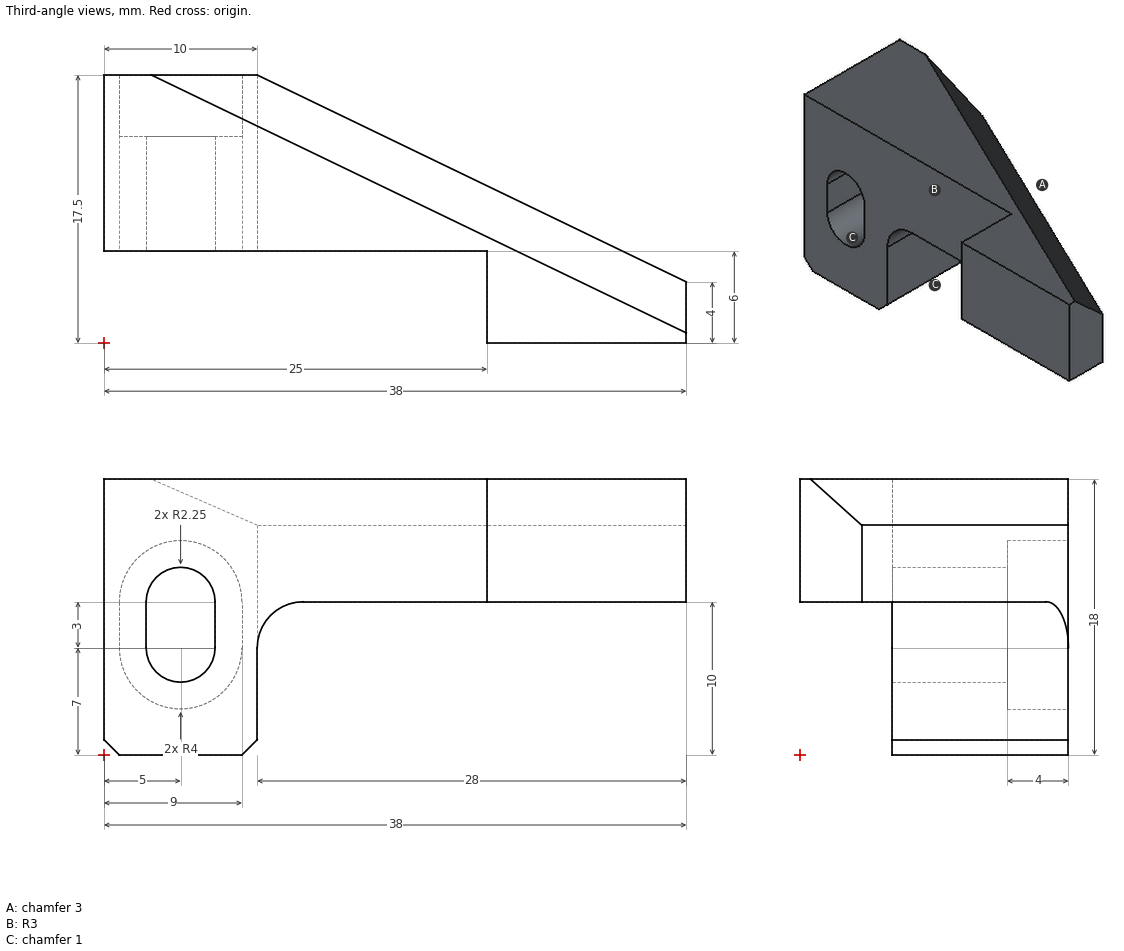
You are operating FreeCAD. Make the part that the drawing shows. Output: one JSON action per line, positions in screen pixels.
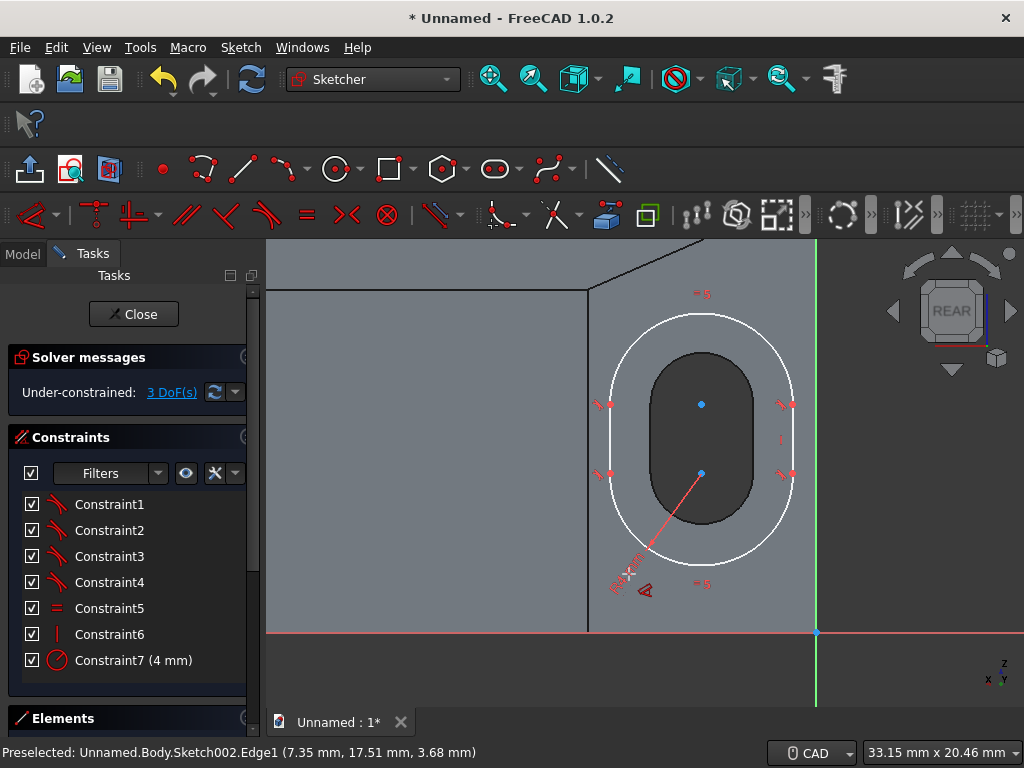
{"action": "left_click", "coordinate": [610, 453]}
{"action": "left_click", "coordinate": [576, 440]}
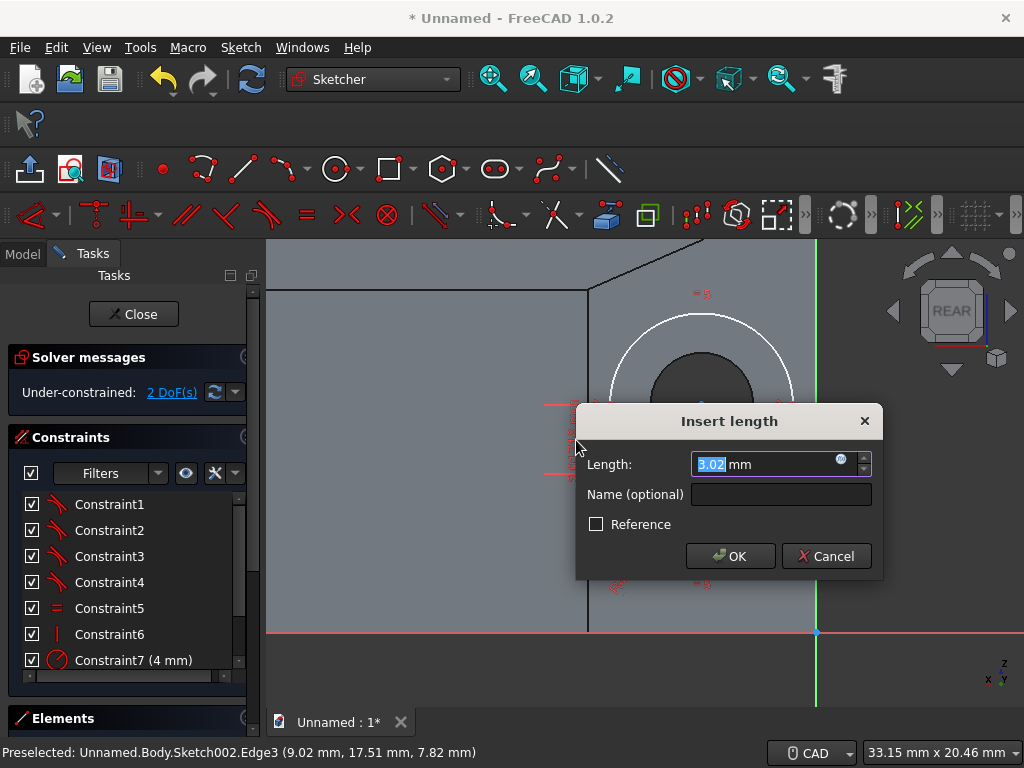
{"action": "type", "text": "3"}
{"action": "key", "text": "Return"}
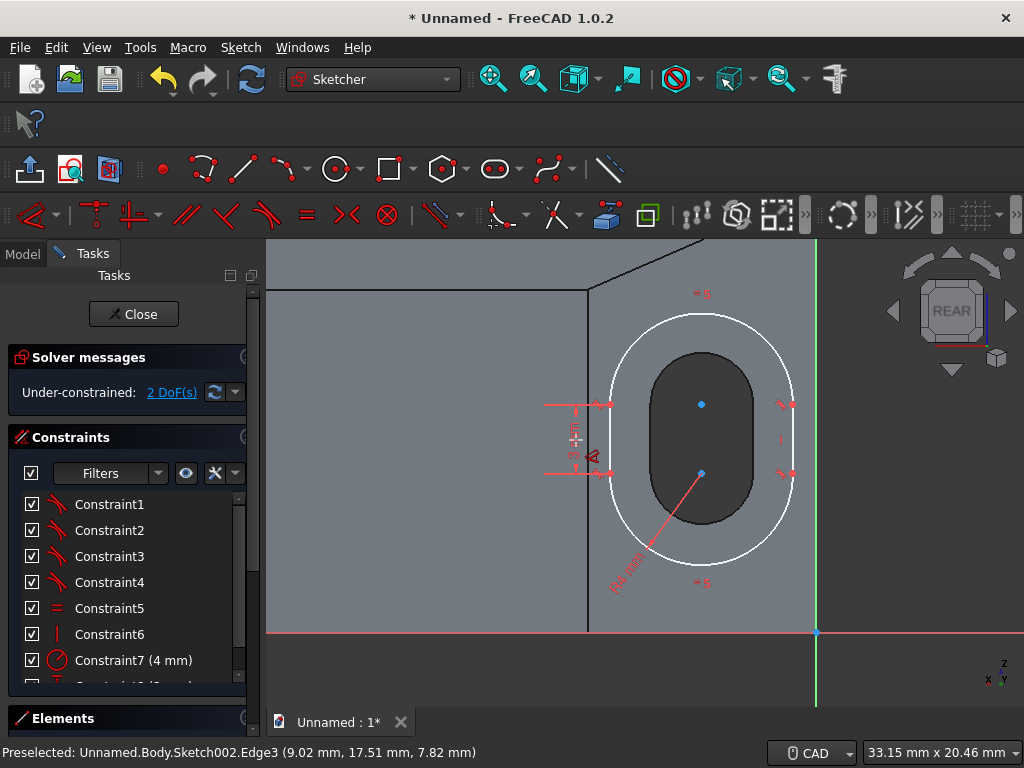
{"action": "left_click", "coordinate": [610, 474]}
{"action": "left_click", "coordinate": [713, 667]}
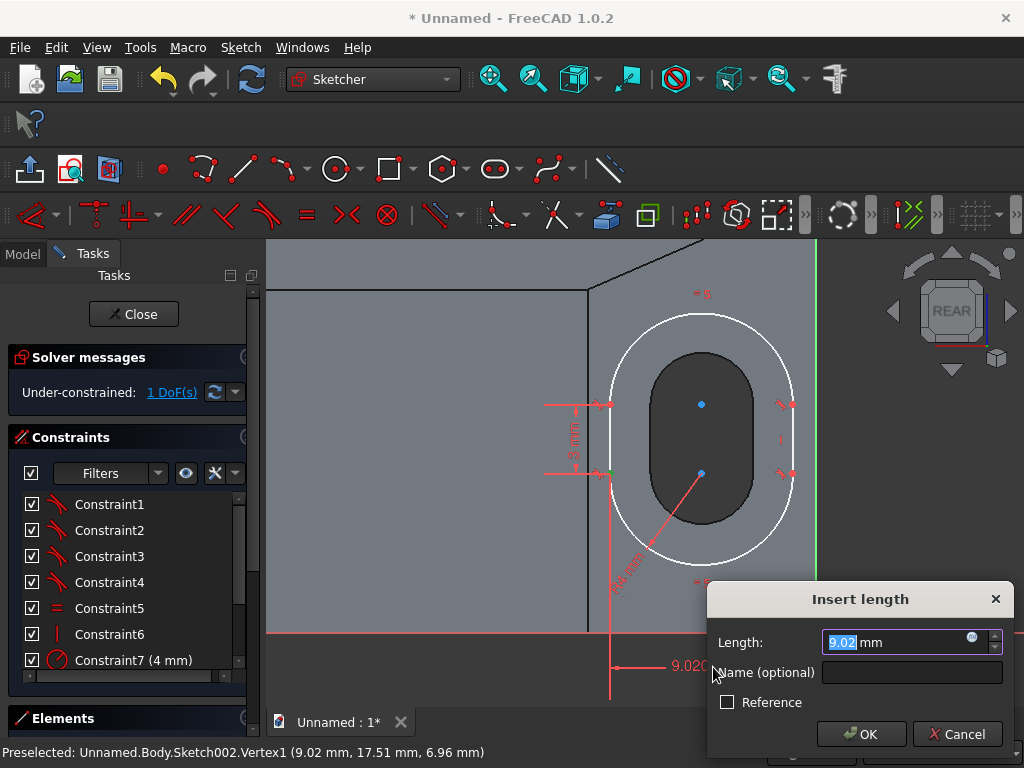
{"action": "type", "text": "9"}
{"action": "key", "text": "Return"}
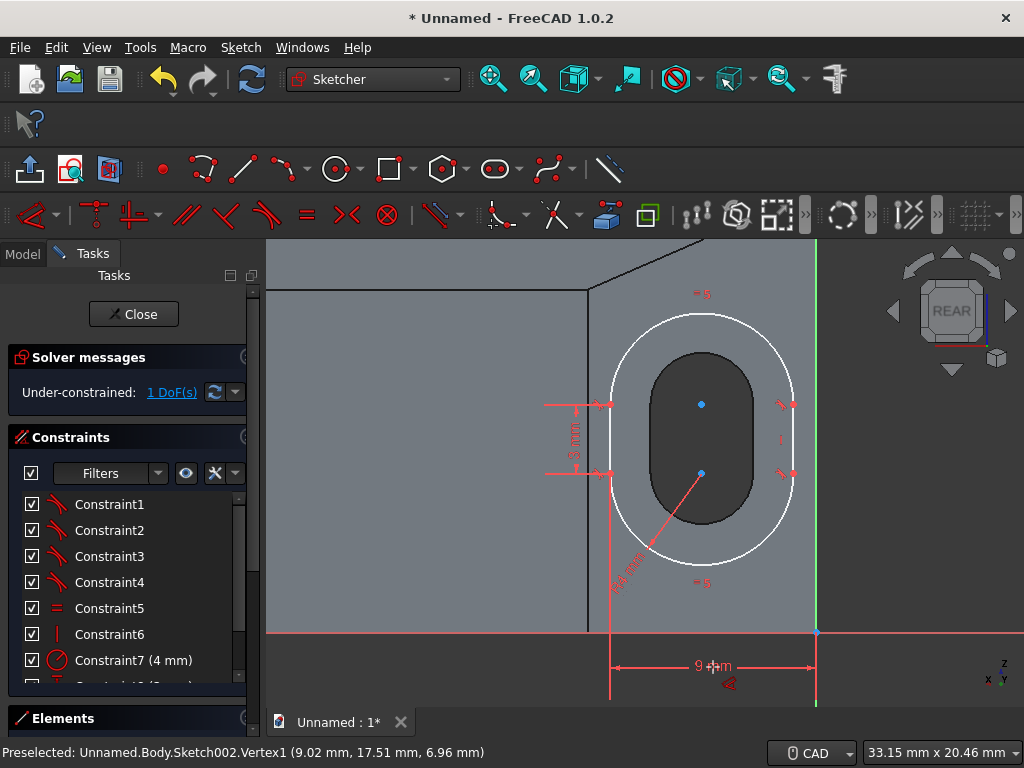
{"action": "left_click", "coordinate": [610, 474]}
{"action": "left_click", "coordinate": [850, 553]}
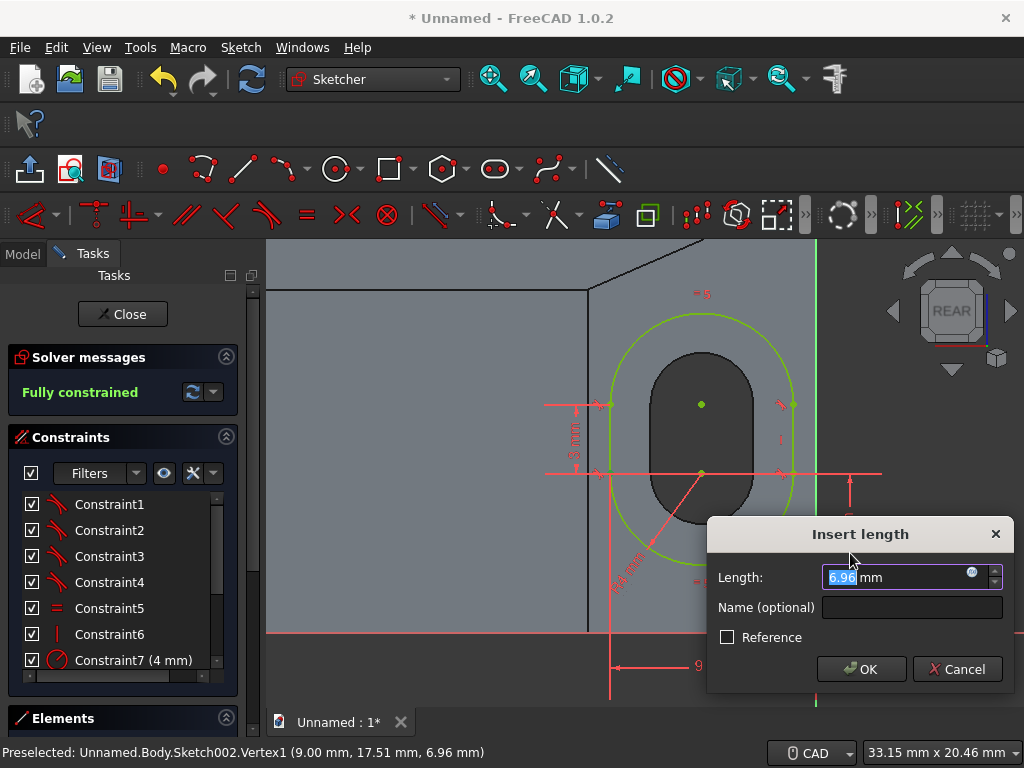
{"action": "type", "text": "7"}
{"action": "key", "text": "Return"}
{"action": "key", "text": "Escape"}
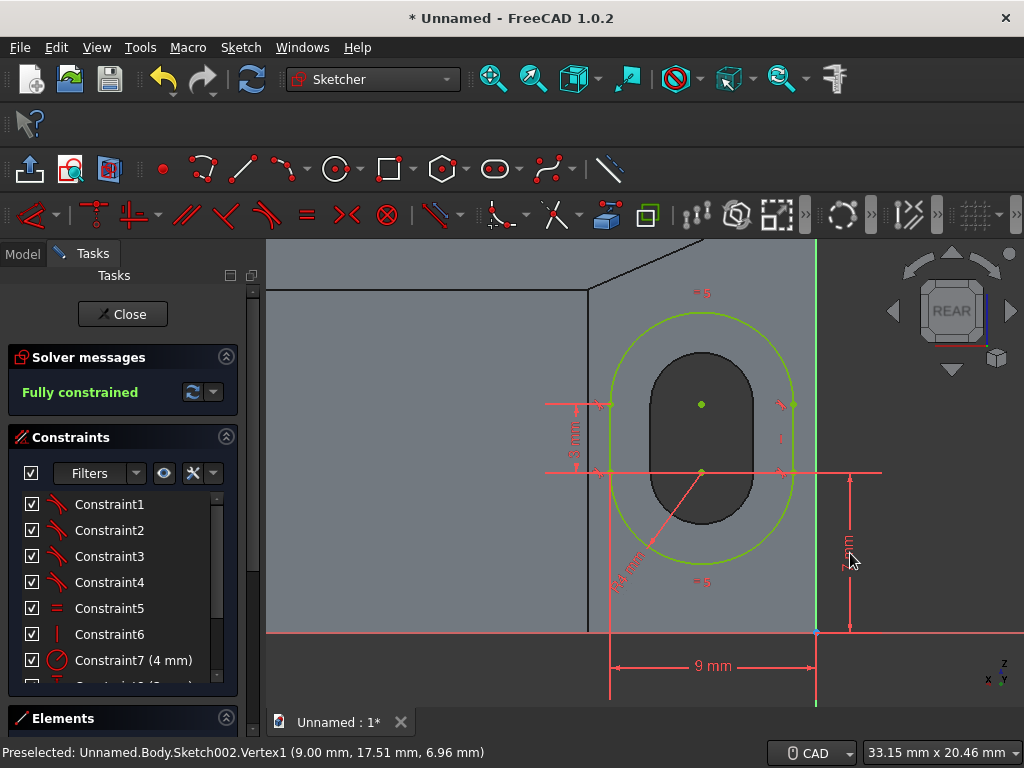
{"action": "left_click", "coordinate": [123, 314]}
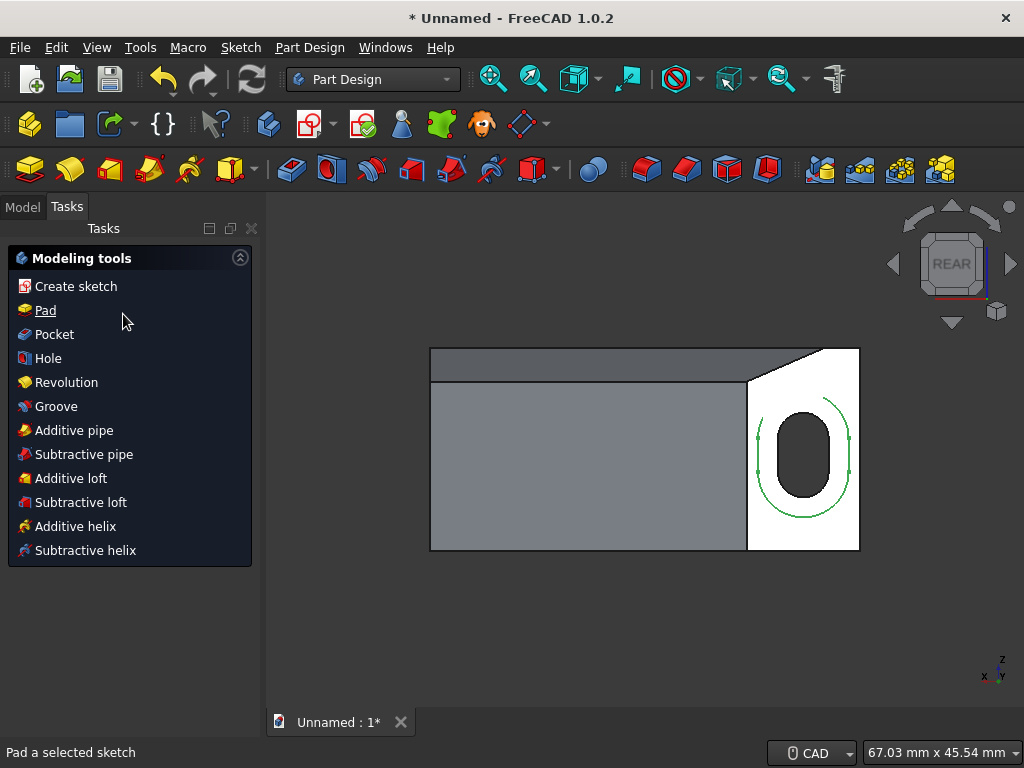
{"action": "left_click", "coordinate": [292, 170]}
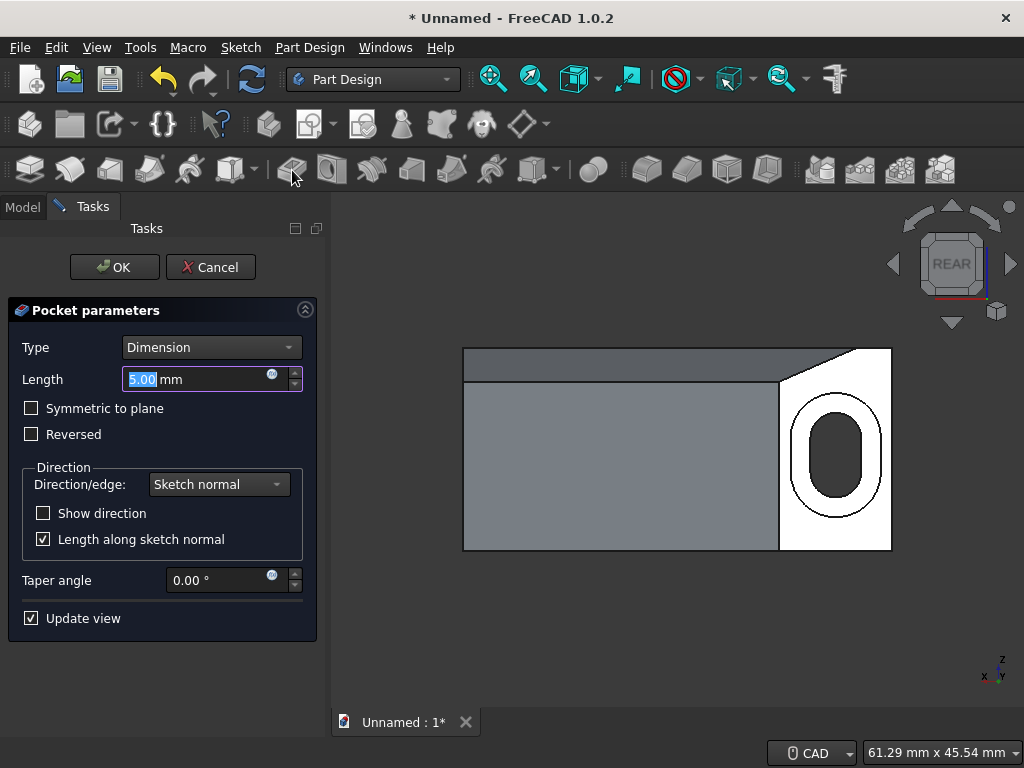
{"action": "type", "text": "4"}
{"action": "key", "text": "Tab"}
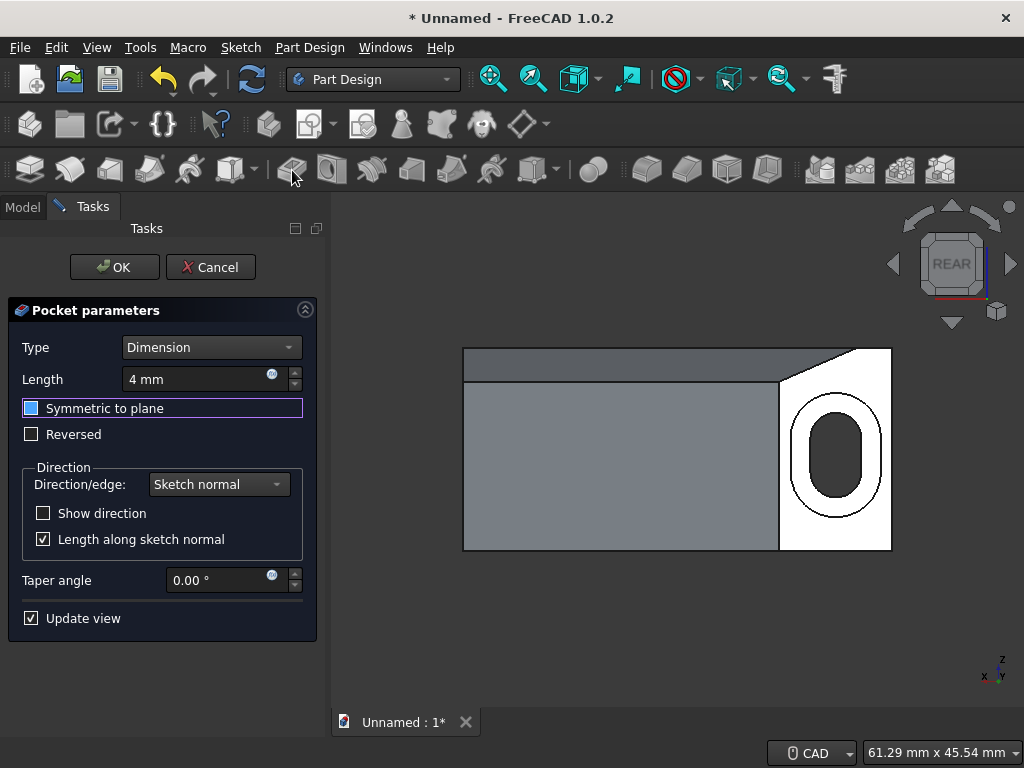
{"action": "left_click", "coordinate": [115, 267]}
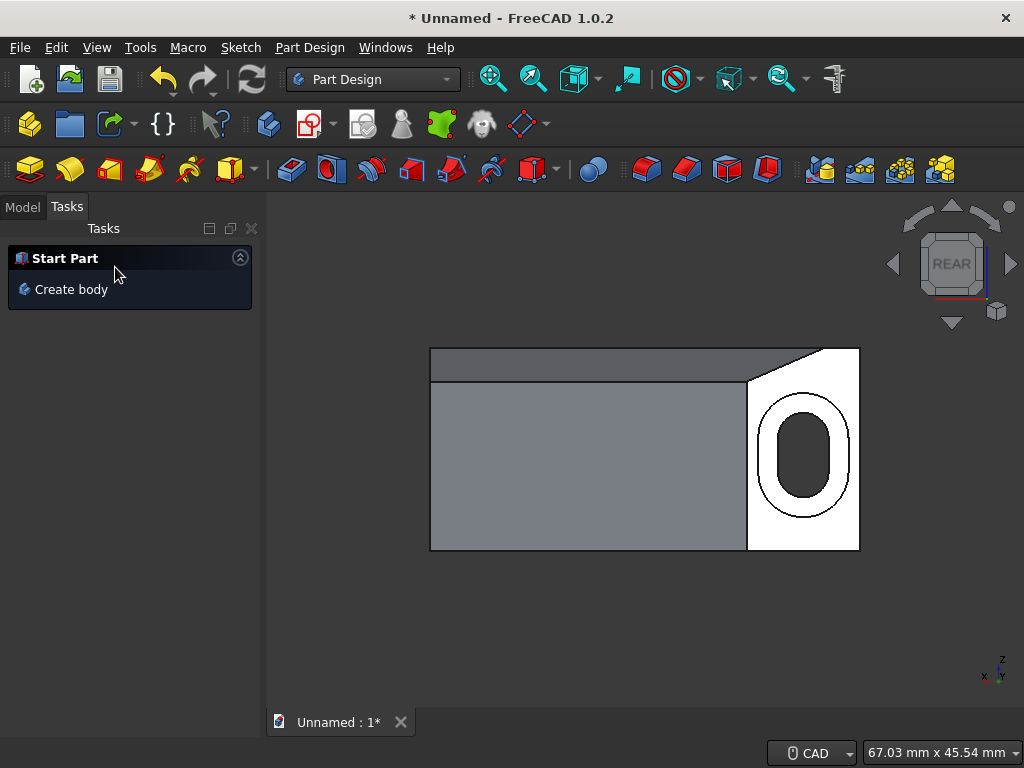
{"action": "key", "text": "0"}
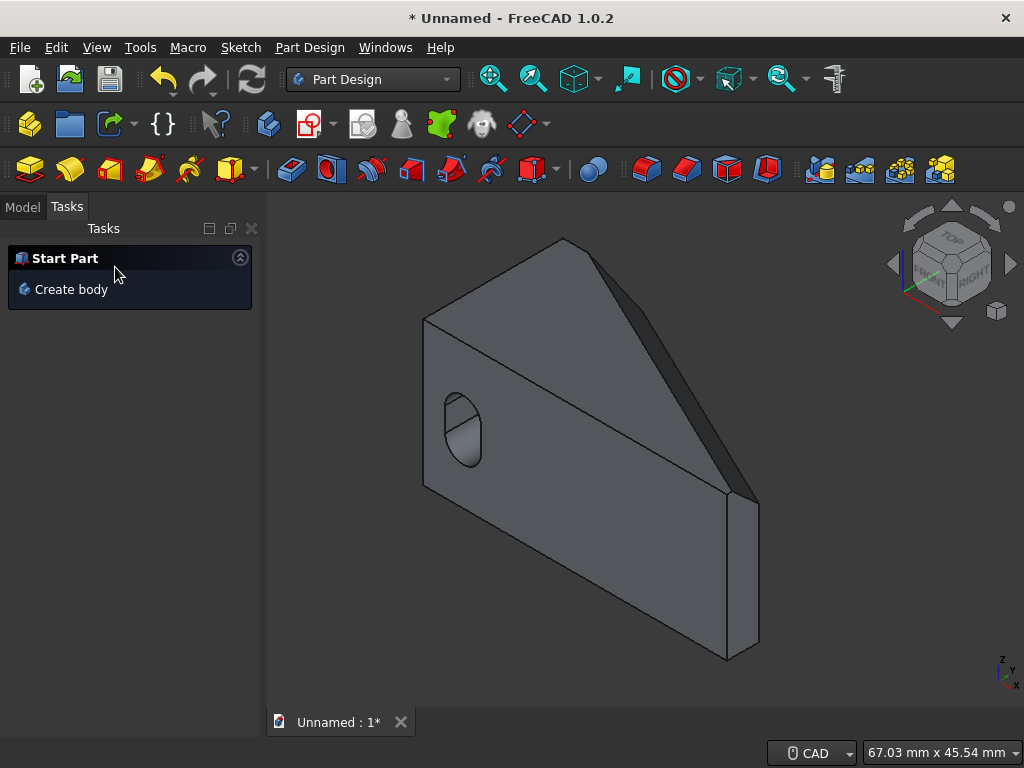
{"action": "left_click", "coordinate": [538, 327]}